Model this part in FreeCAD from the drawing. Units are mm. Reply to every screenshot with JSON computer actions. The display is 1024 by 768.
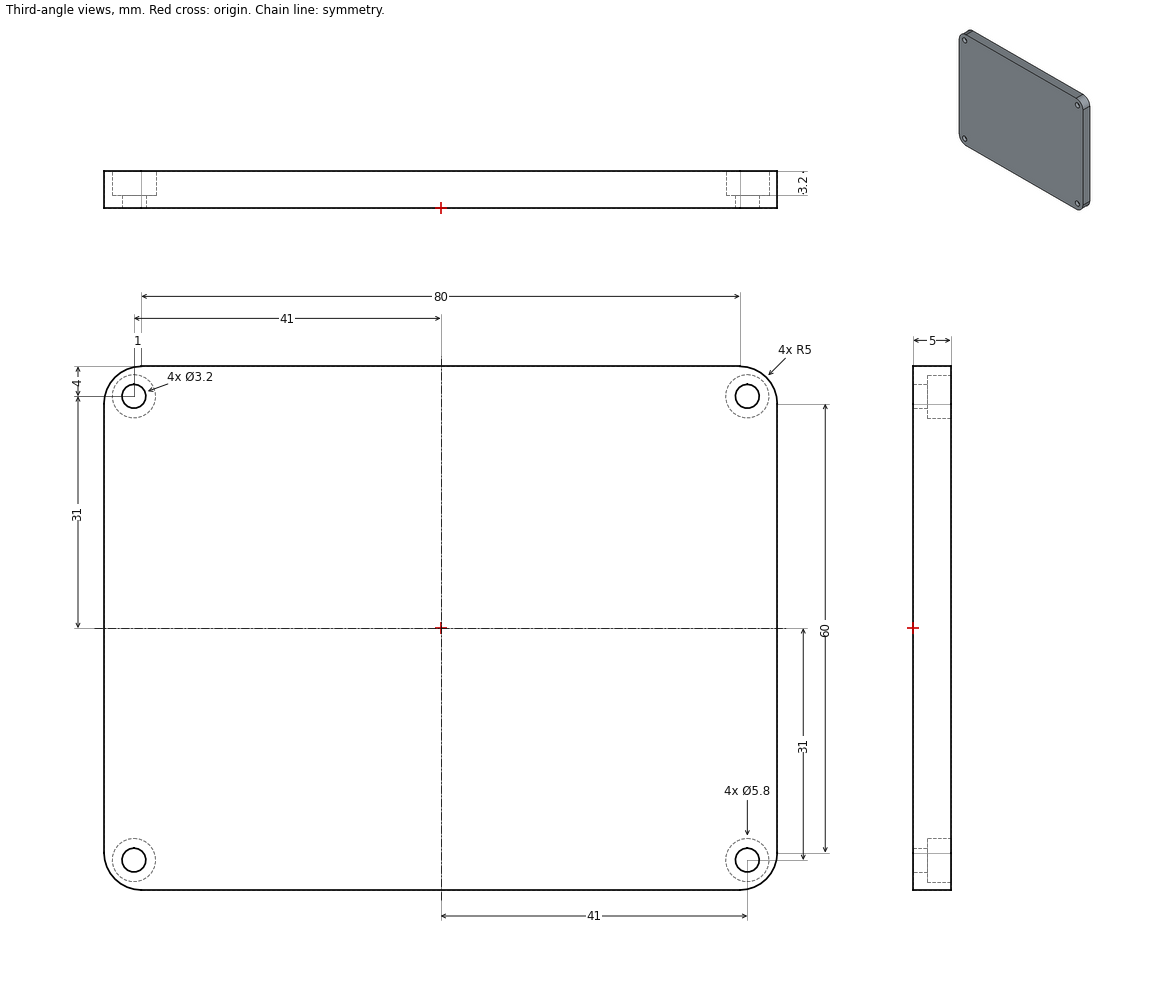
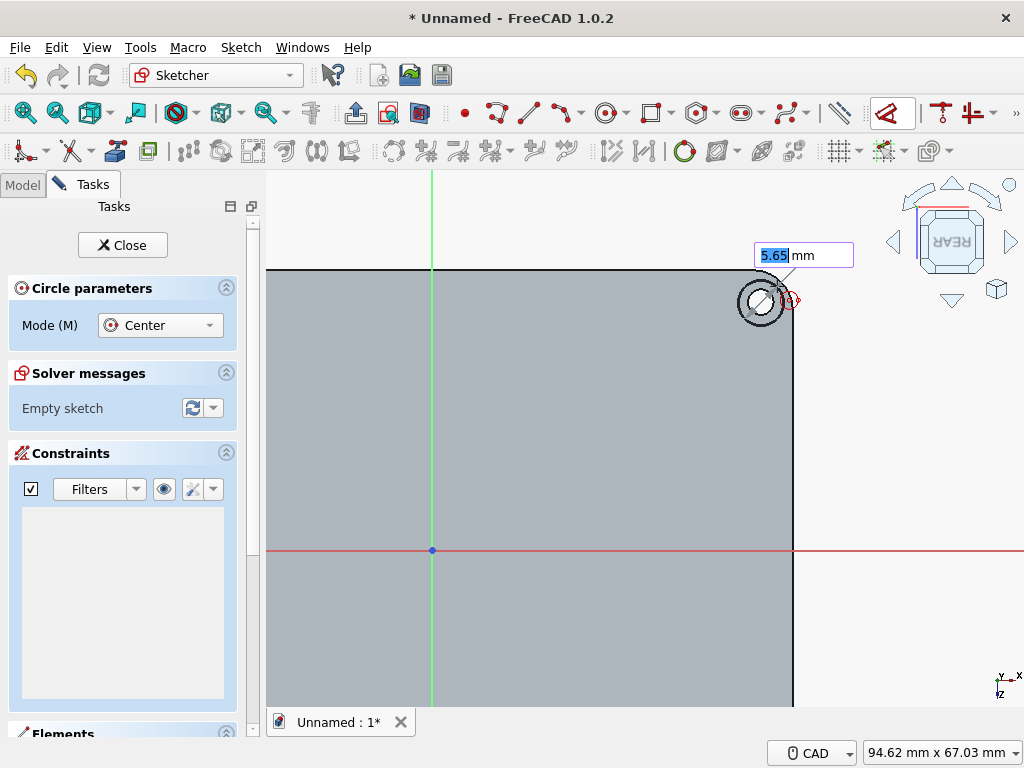
{"action": "type", "text": "5.8"}
{"action": "key", "text": "Return"}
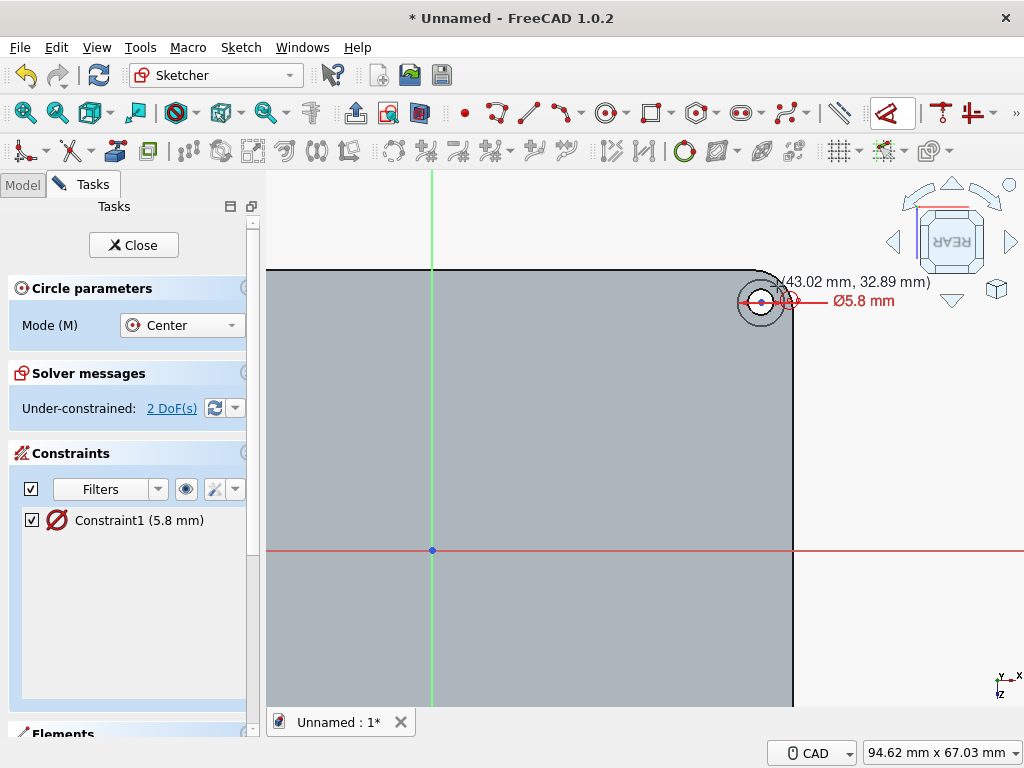
{"action": "scroll", "coordinate": [752, 302], "scroll_direction": "down", "scroll_amount": 3}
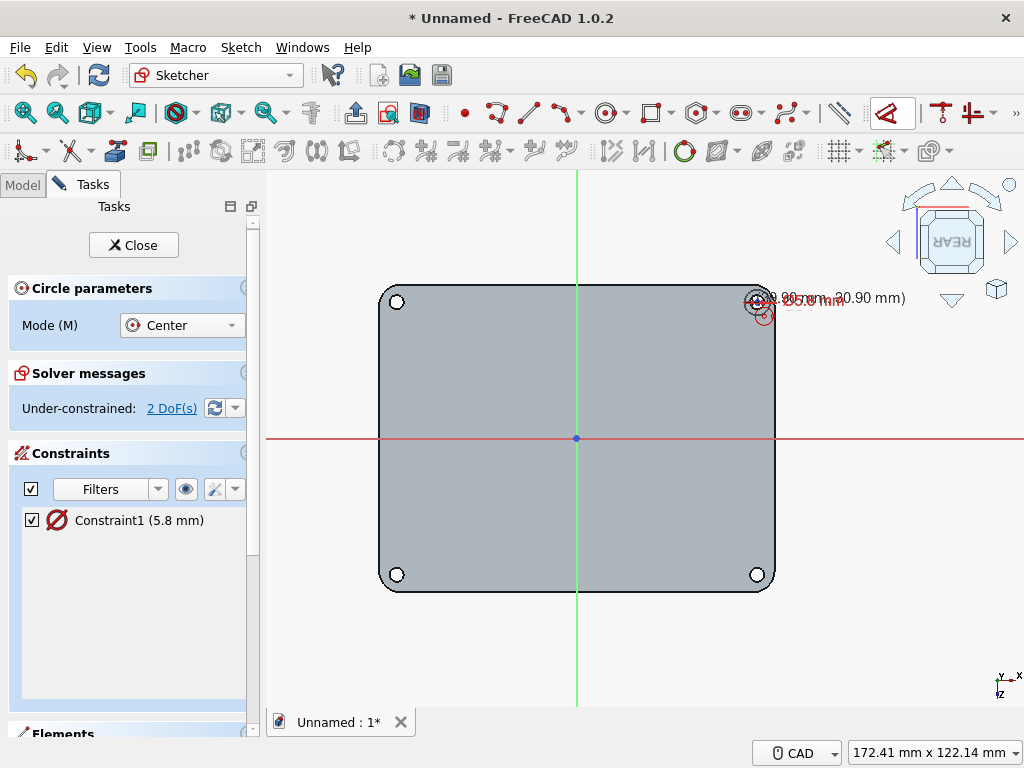
{"action": "scroll", "coordinate": [397, 302], "scroll_direction": "up", "scroll_amount": 3}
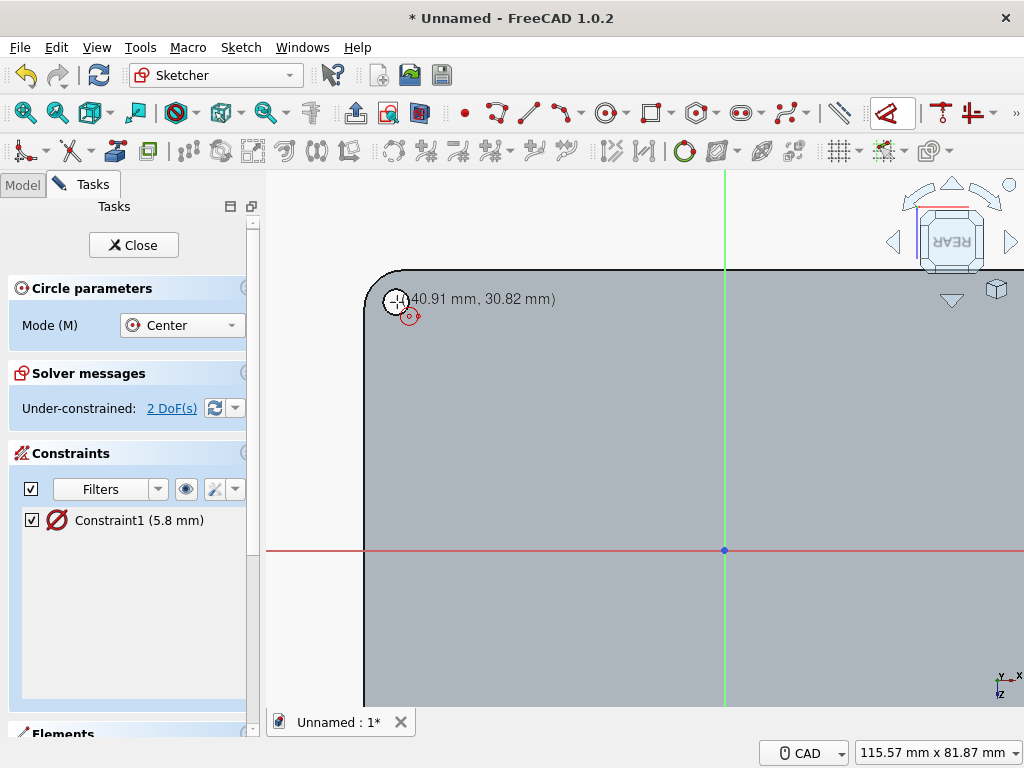
{"action": "left_click", "coordinate": [396, 302]}
{"action": "mouse_move", "coordinate": [413, 286]}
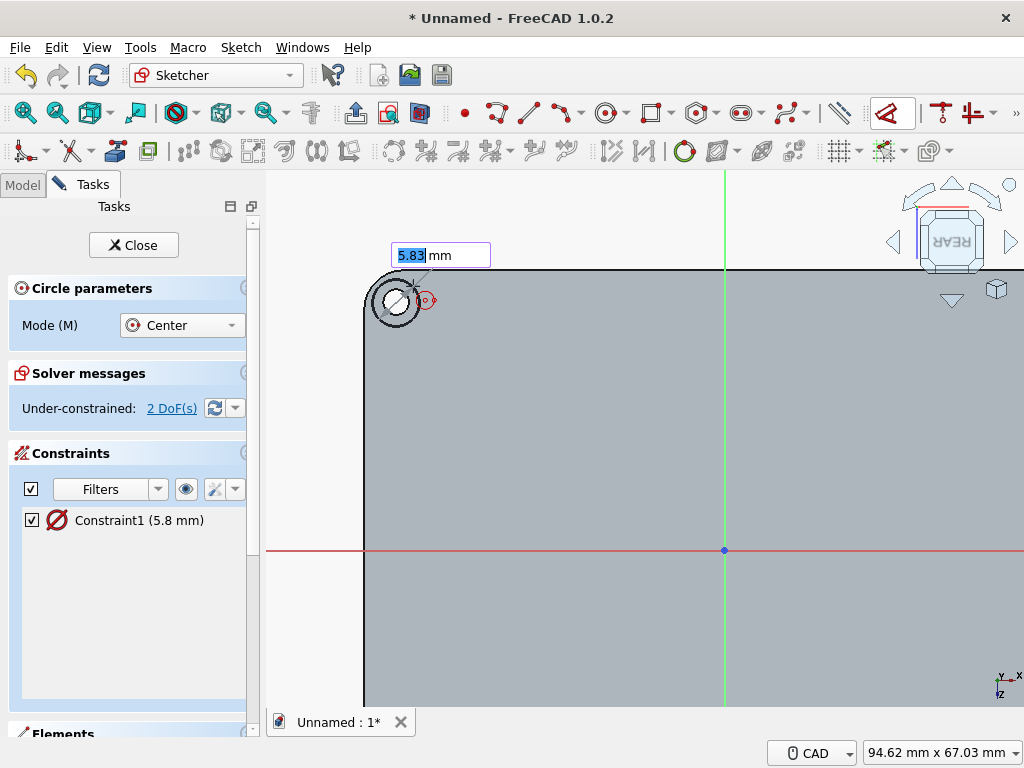
{"action": "type", "text": "5.8"}
{"action": "key", "text": "Return"}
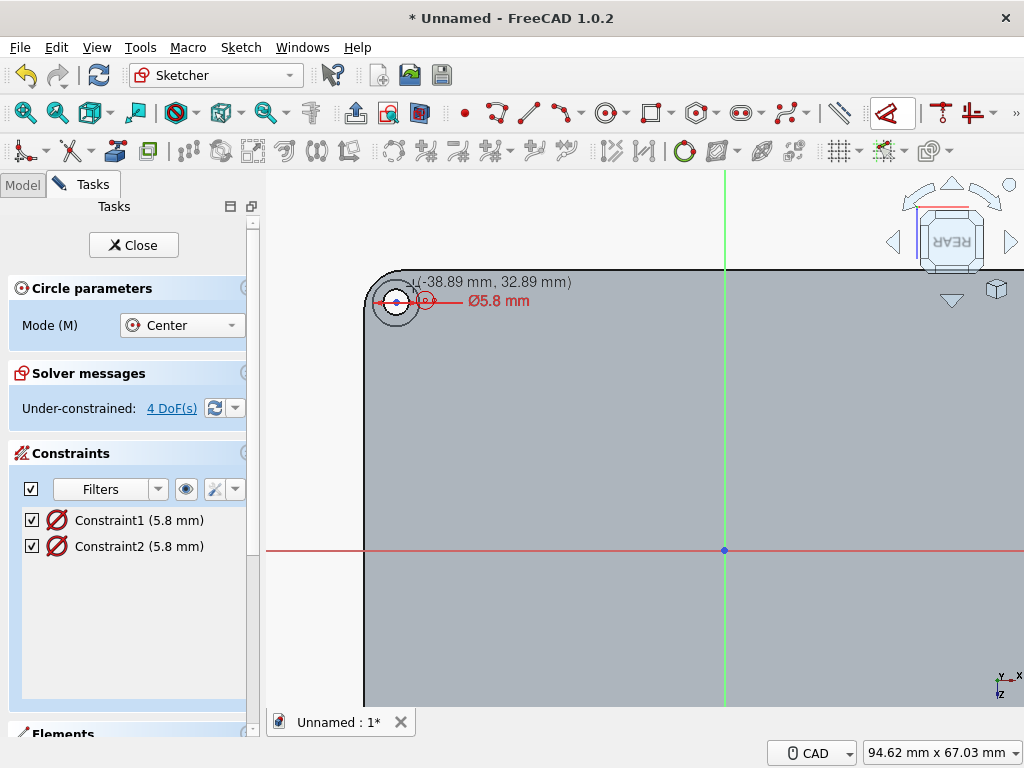
{"action": "scroll", "coordinate": [396, 302], "scroll_direction": "down", "scroll_amount": 3}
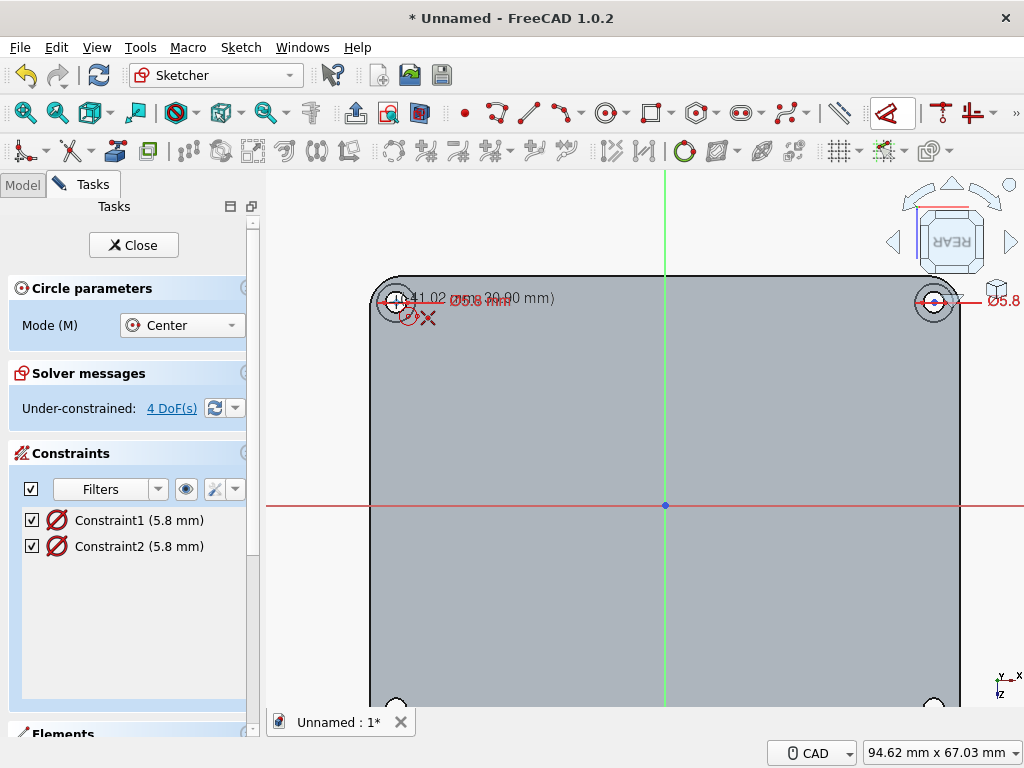
{"action": "scroll", "coordinate": [396, 575], "scroll_direction": "up", "scroll_amount": 3}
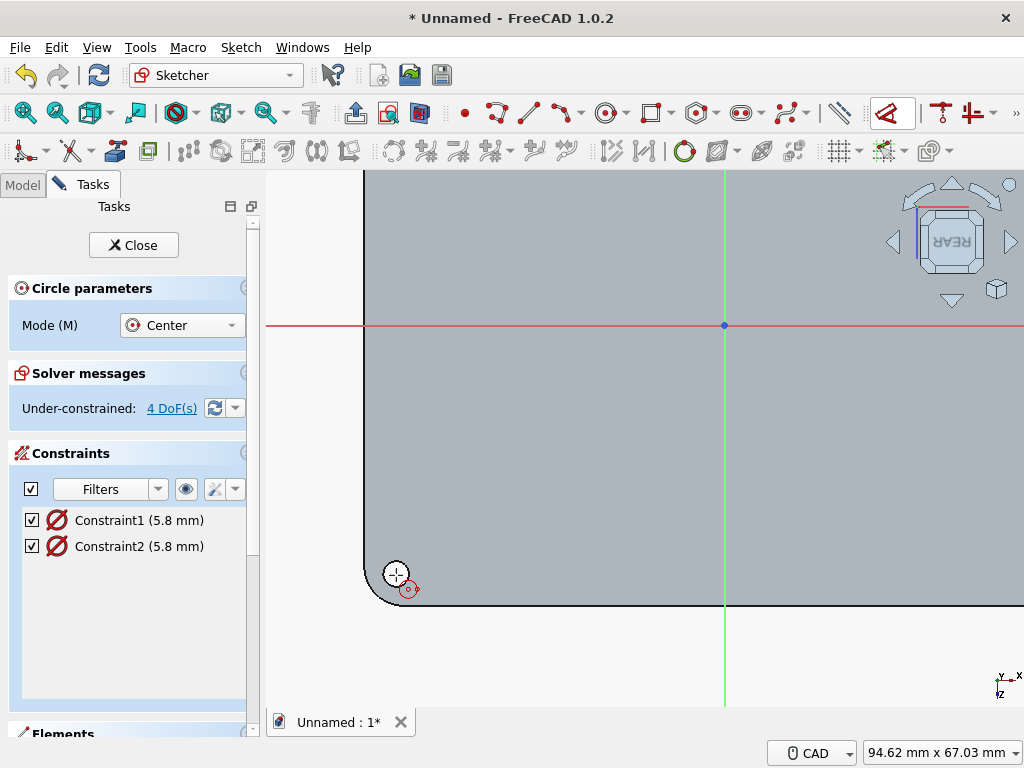
{"action": "left_click", "coordinate": [396, 574]}
{"action": "mouse_move", "coordinate": [413, 558]}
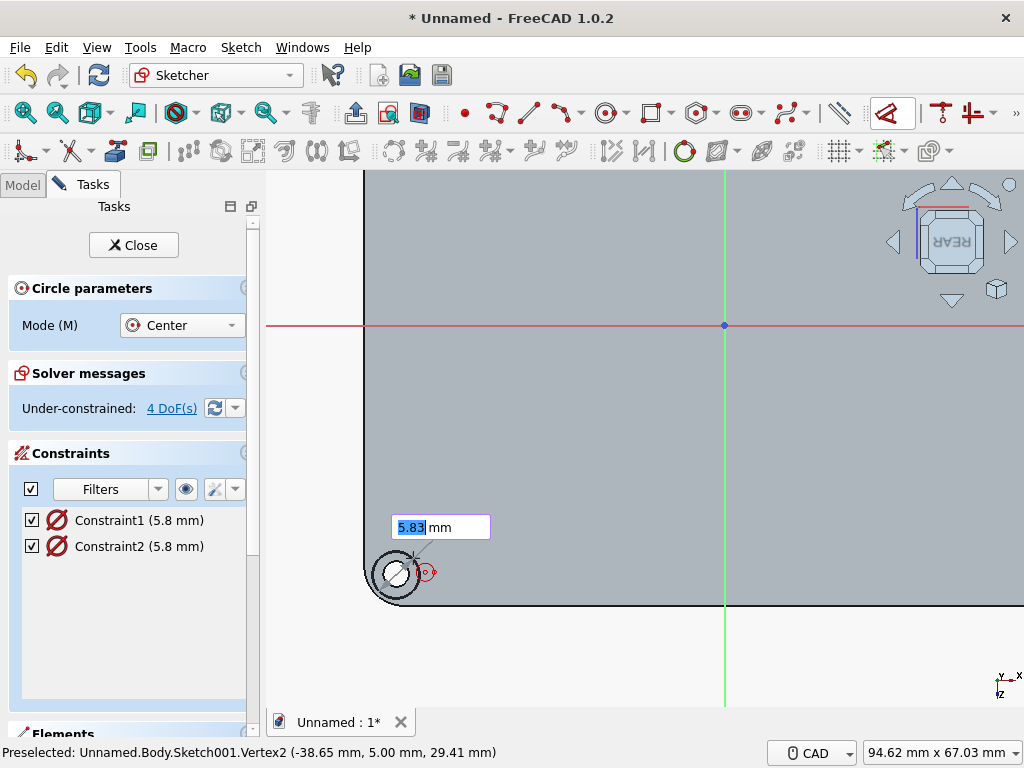
{"action": "type", "text": "5.8"}
{"action": "key", "text": "Return"}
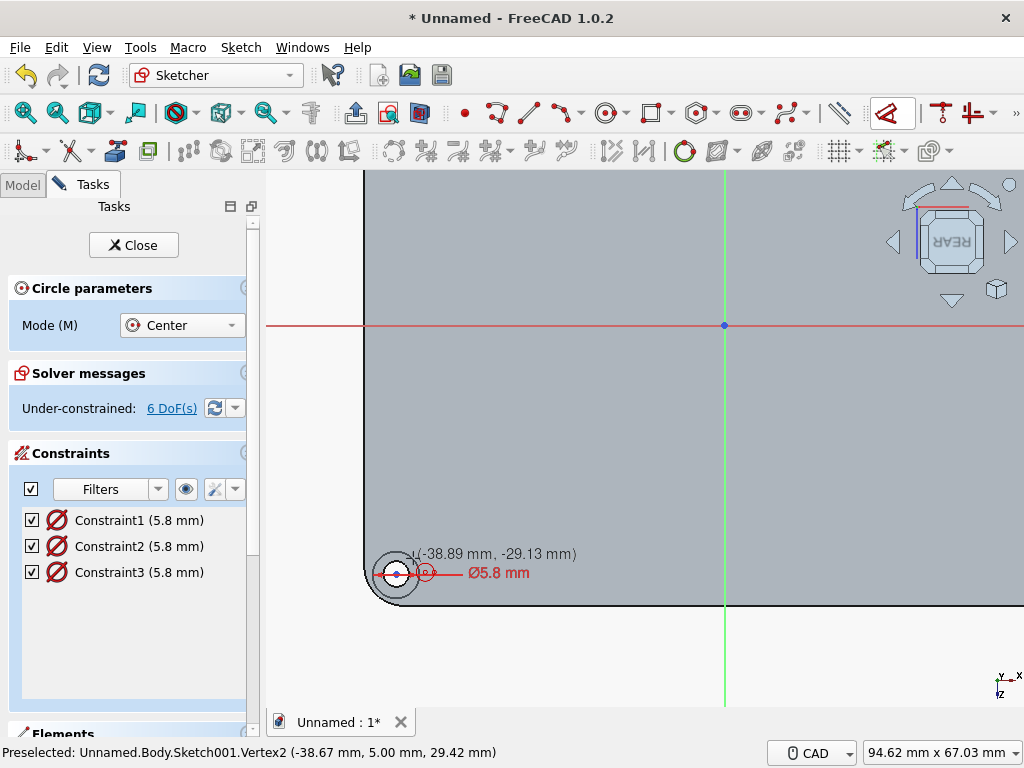
{"action": "scroll", "coordinate": [396, 576], "scroll_direction": "down", "scroll_amount": 3}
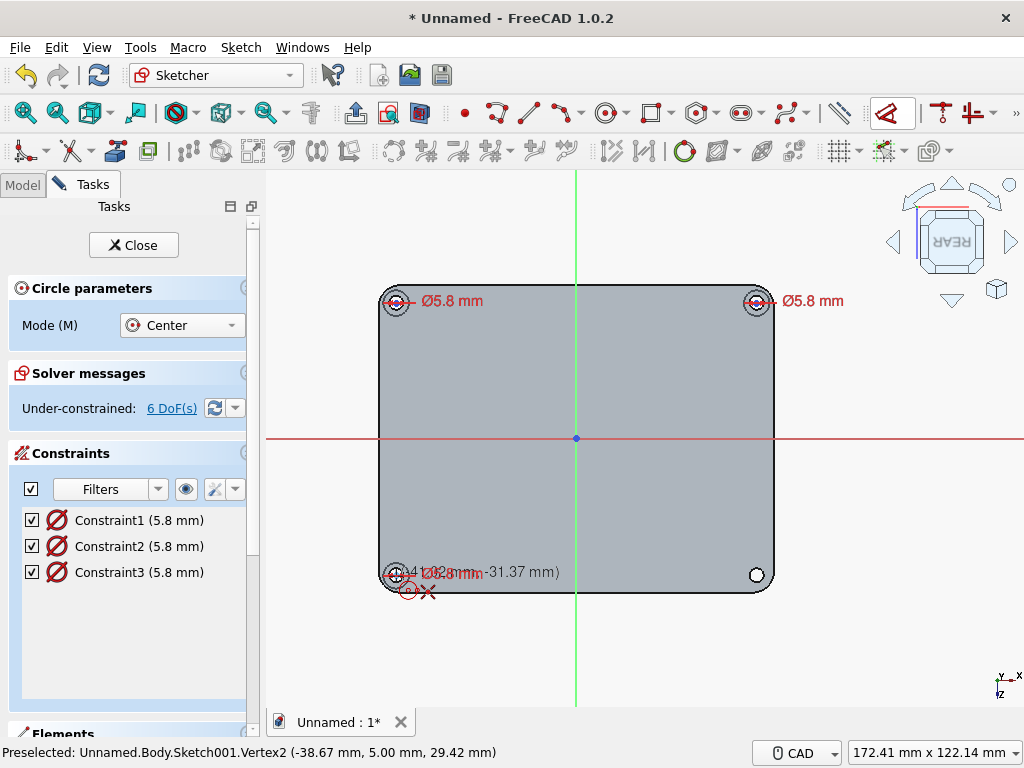
{"action": "scroll", "coordinate": [757, 575], "scroll_direction": "up", "scroll_amount": 3}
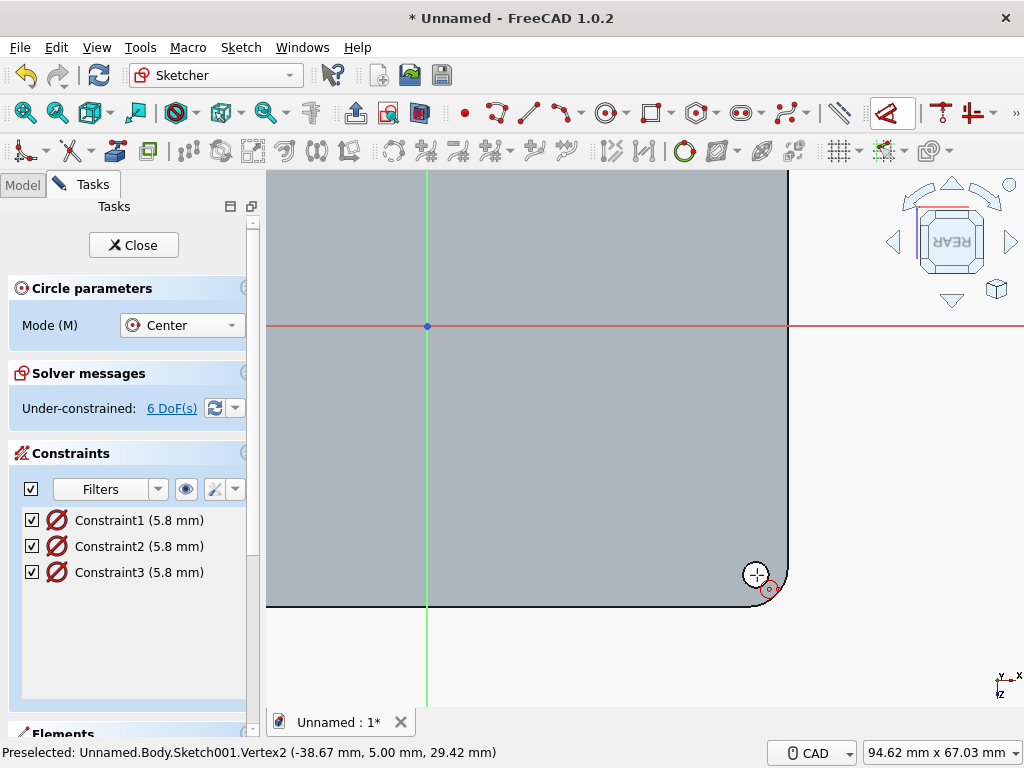
{"action": "left_click", "coordinate": [756, 575]}
{"action": "mouse_move", "coordinate": [772, 558]}